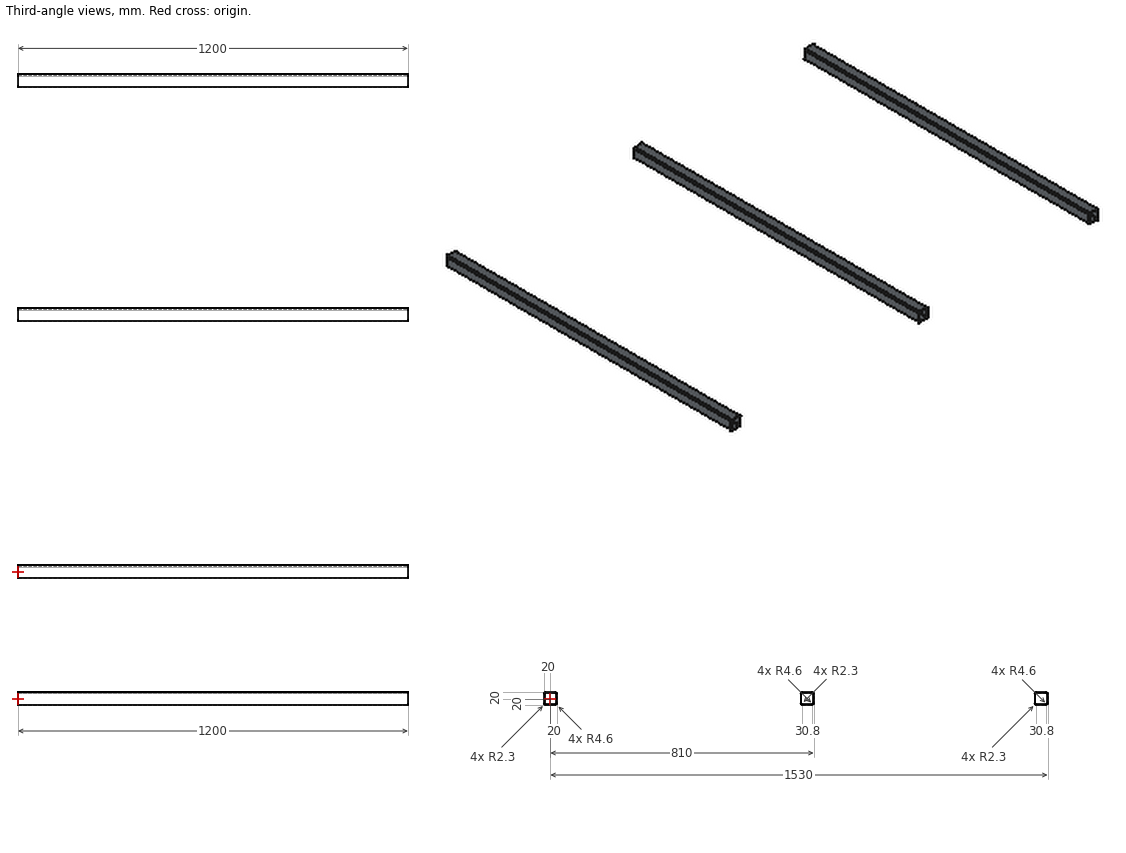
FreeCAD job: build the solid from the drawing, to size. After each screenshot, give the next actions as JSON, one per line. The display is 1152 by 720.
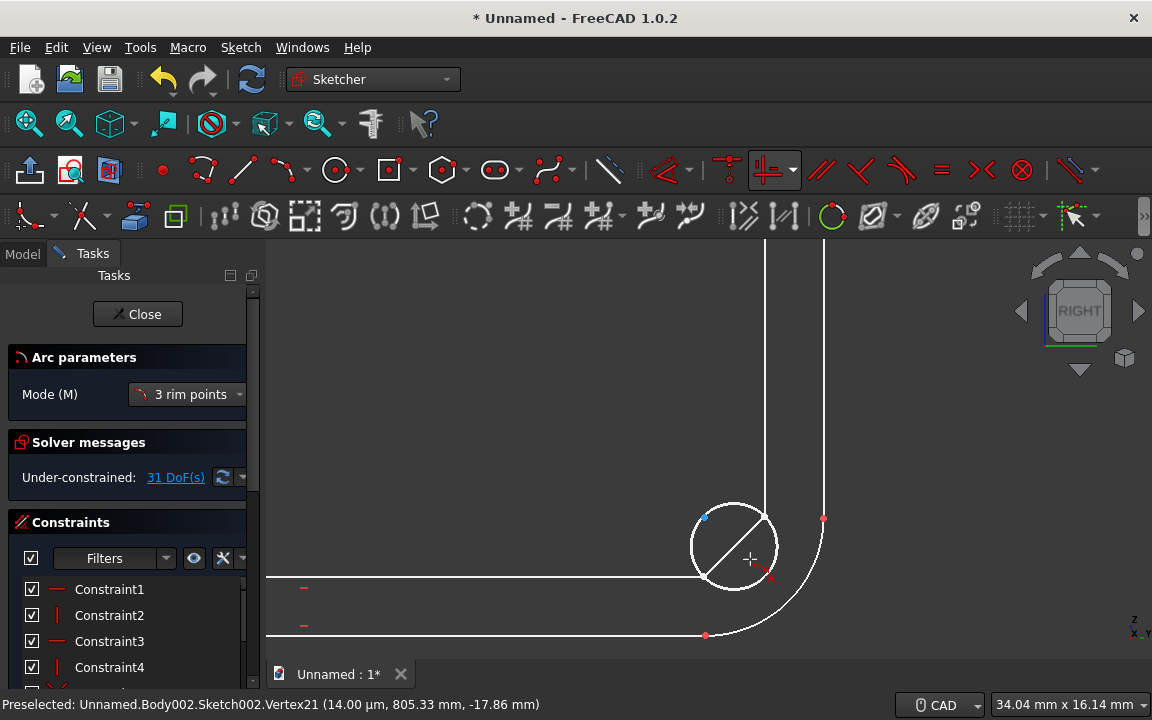
{"action": "left_click", "coordinate": [748, 555]}
{"action": "key", "text": "Escape"}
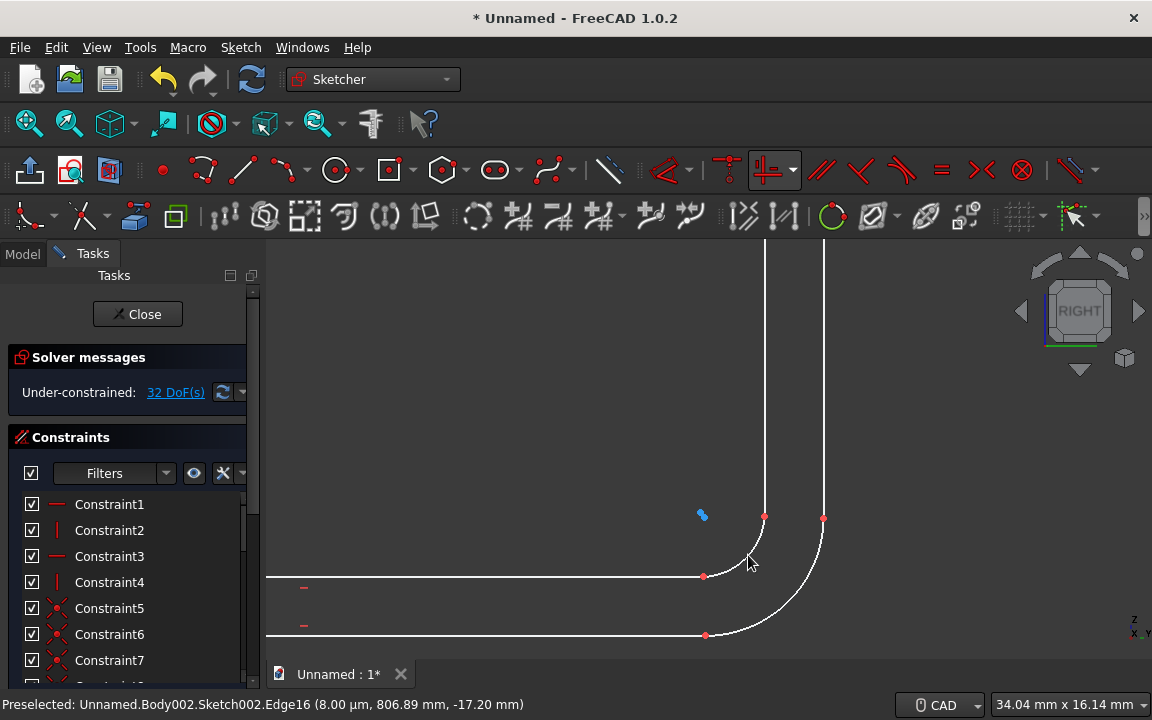
{"action": "scroll", "coordinate": [750, 559], "scroll_direction": "down", "scroll_amount": 7}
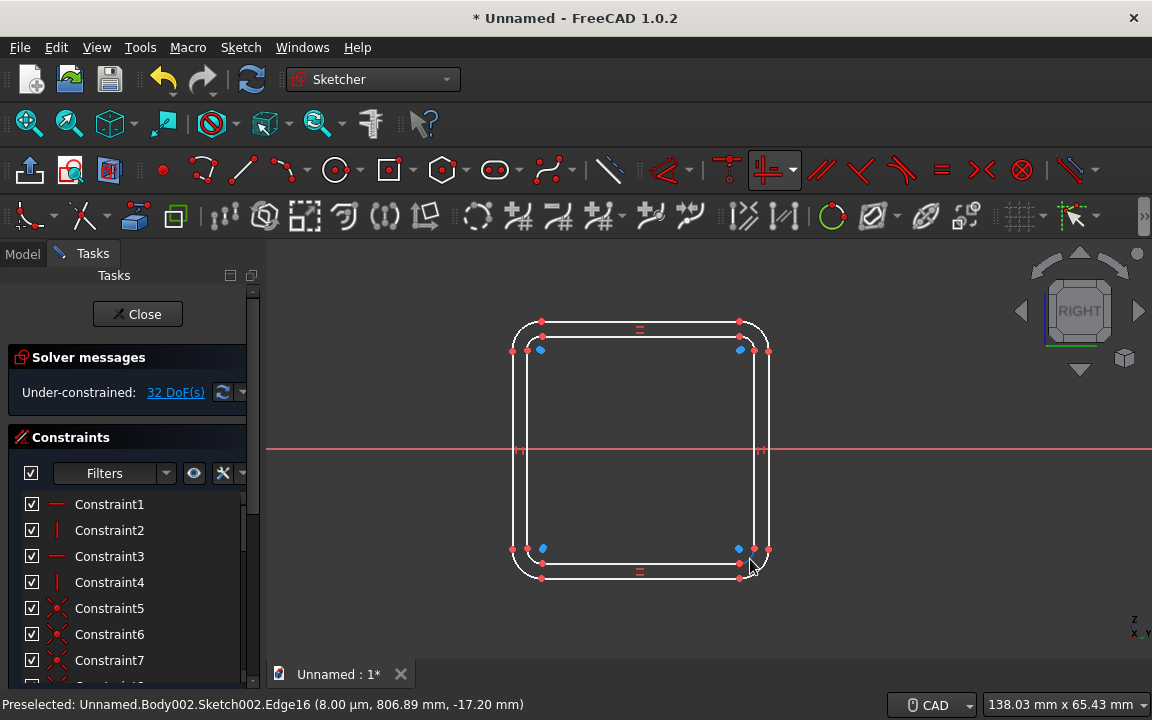
{"action": "left_click", "coordinate": [601, 579]}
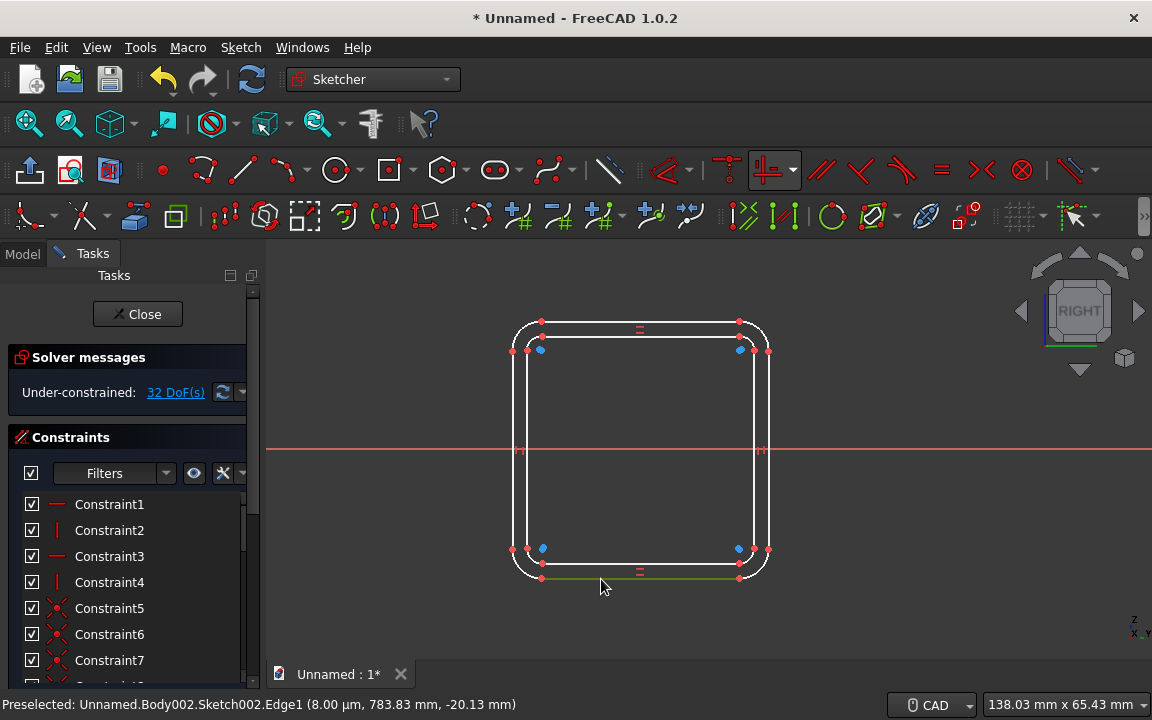
{"action": "left_click", "coordinate": [753, 575]}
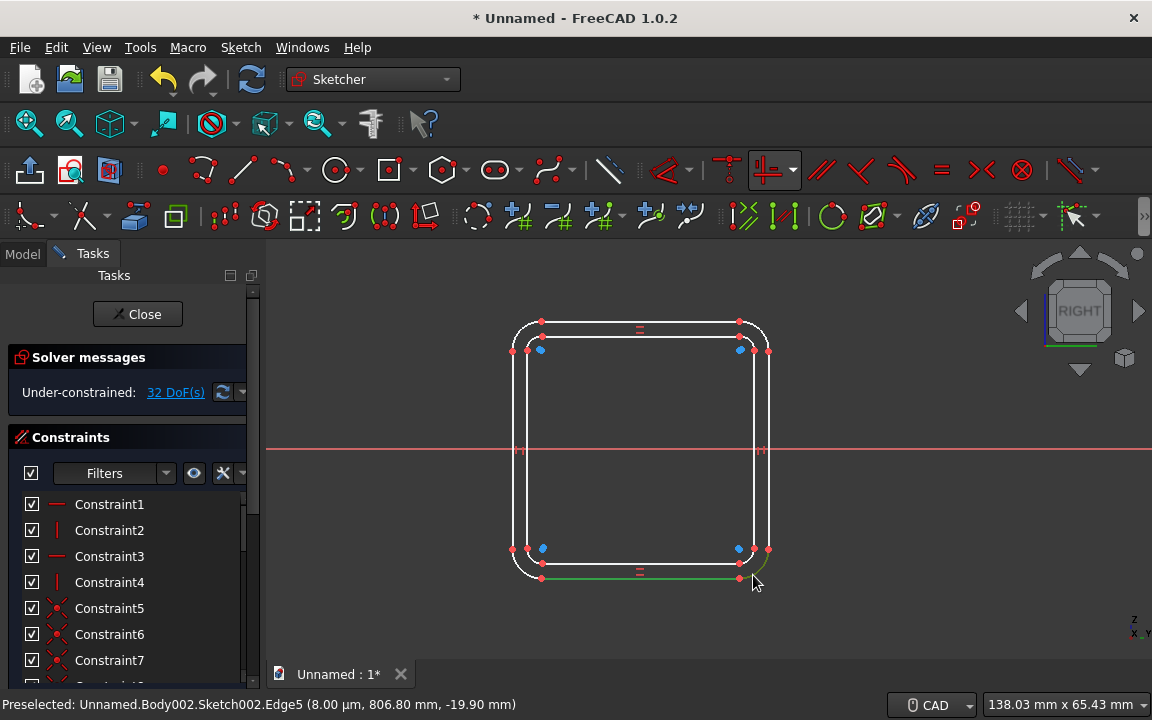
{"action": "left_click", "coordinate": [902, 170]}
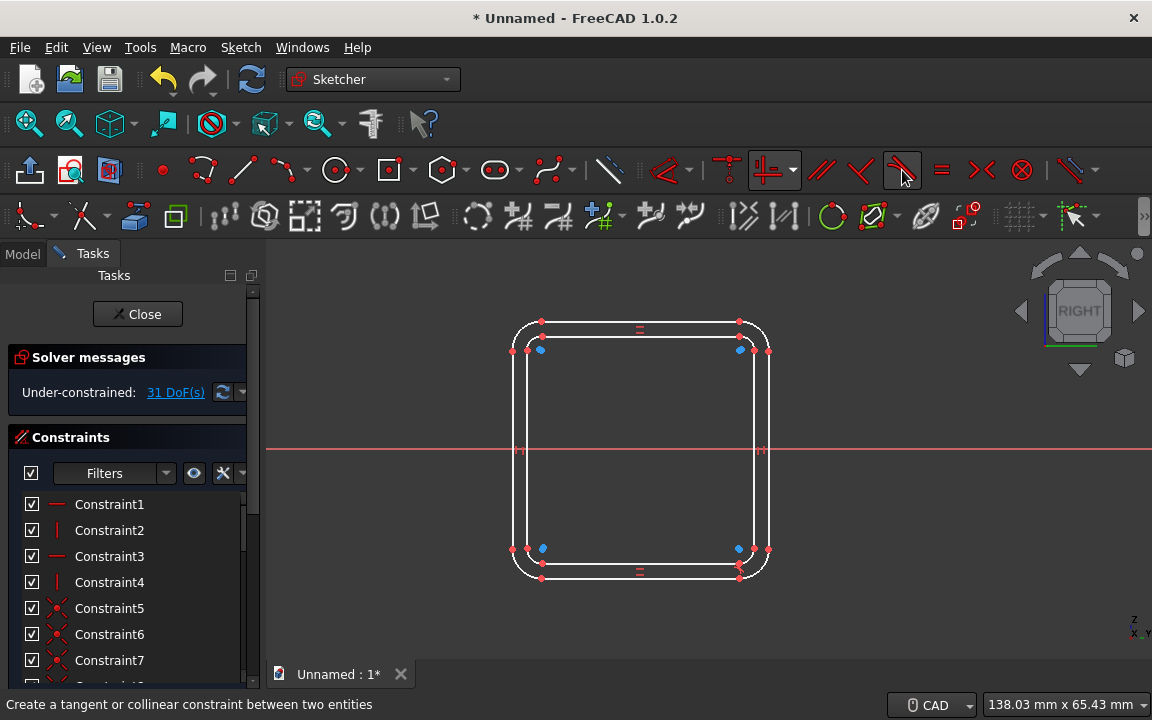
{"action": "left_click", "coordinate": [601, 579]}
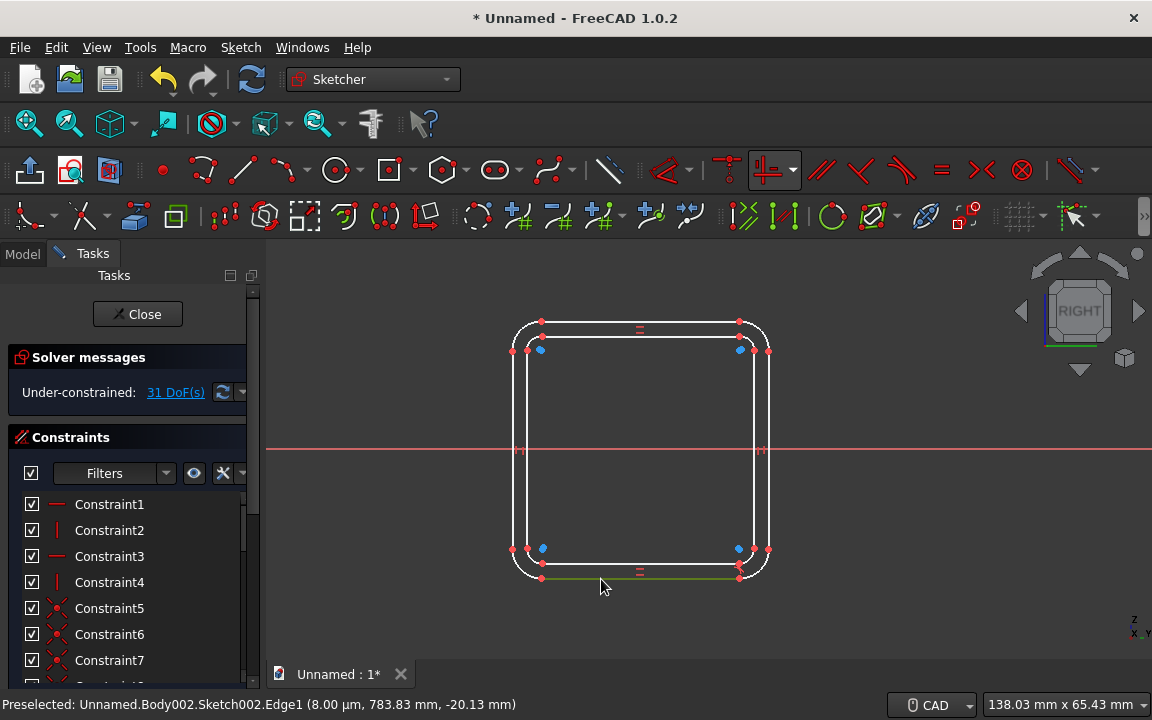
{"action": "left_click", "coordinate": [516, 563]}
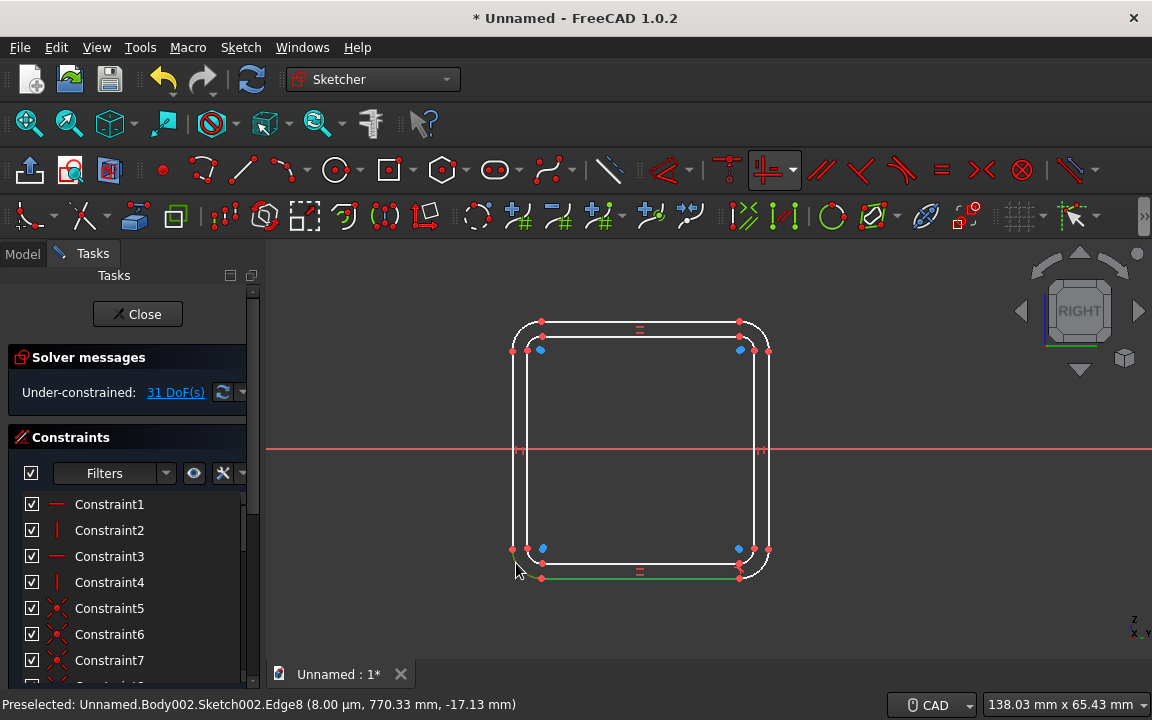
{"action": "key", "text": "t"}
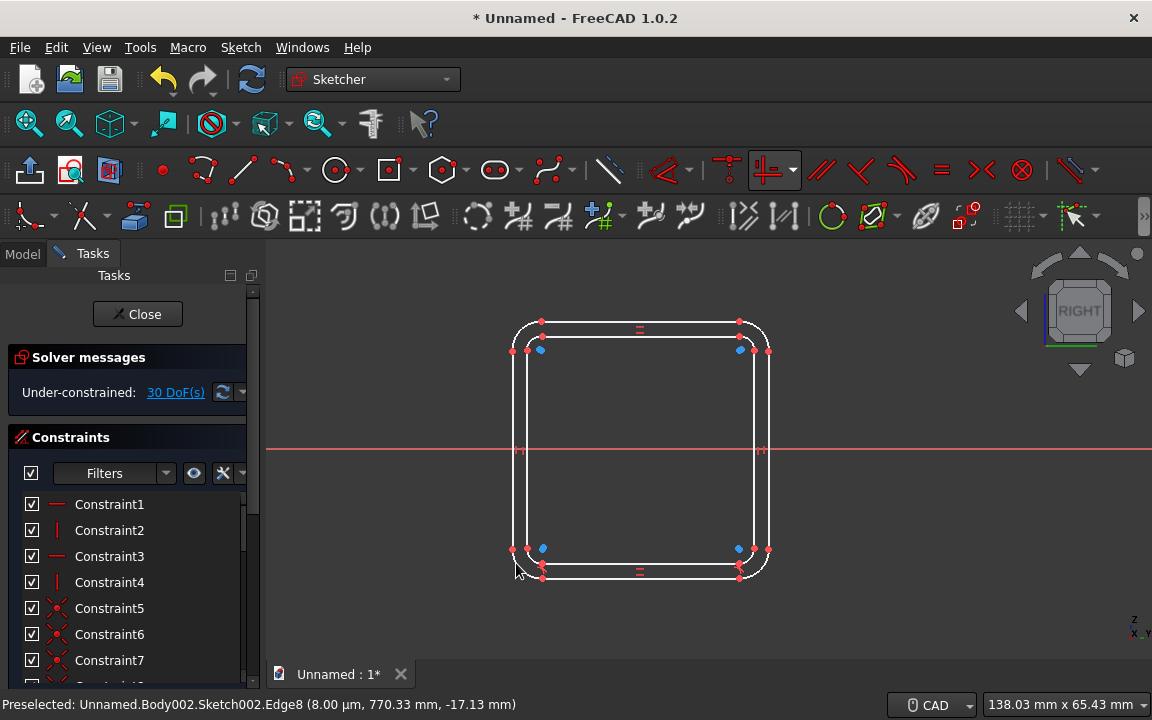
{"action": "left_click", "coordinate": [769, 490]}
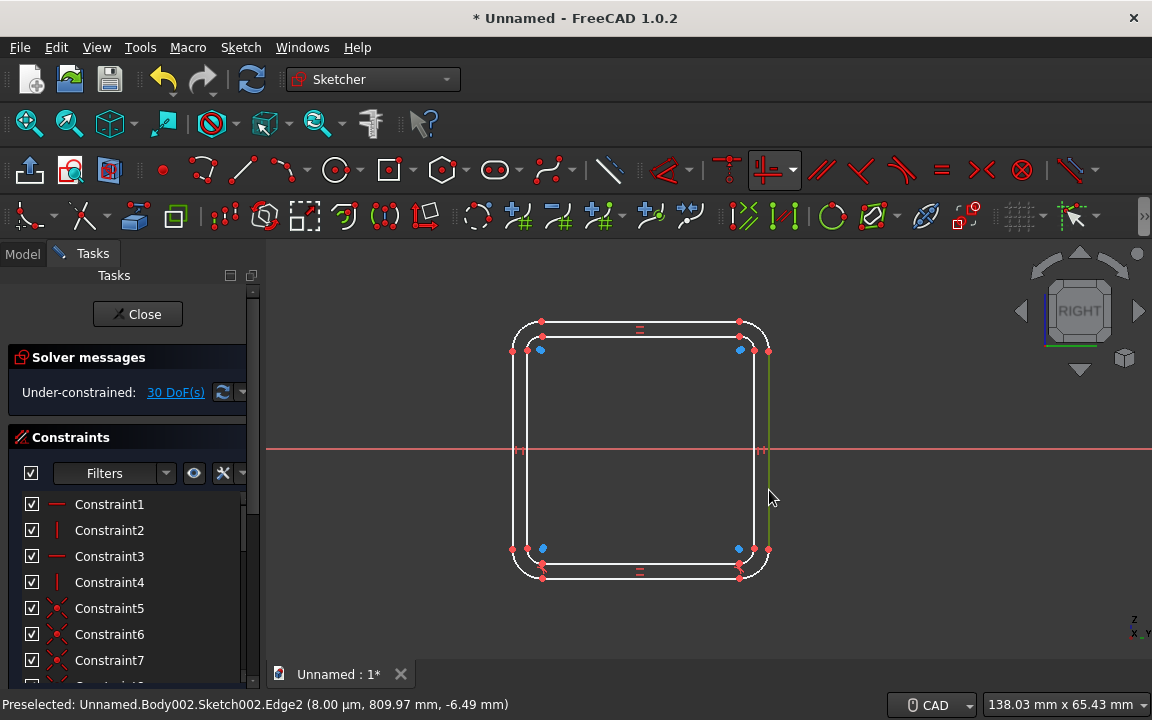
{"action": "left_click", "coordinate": [753, 575]}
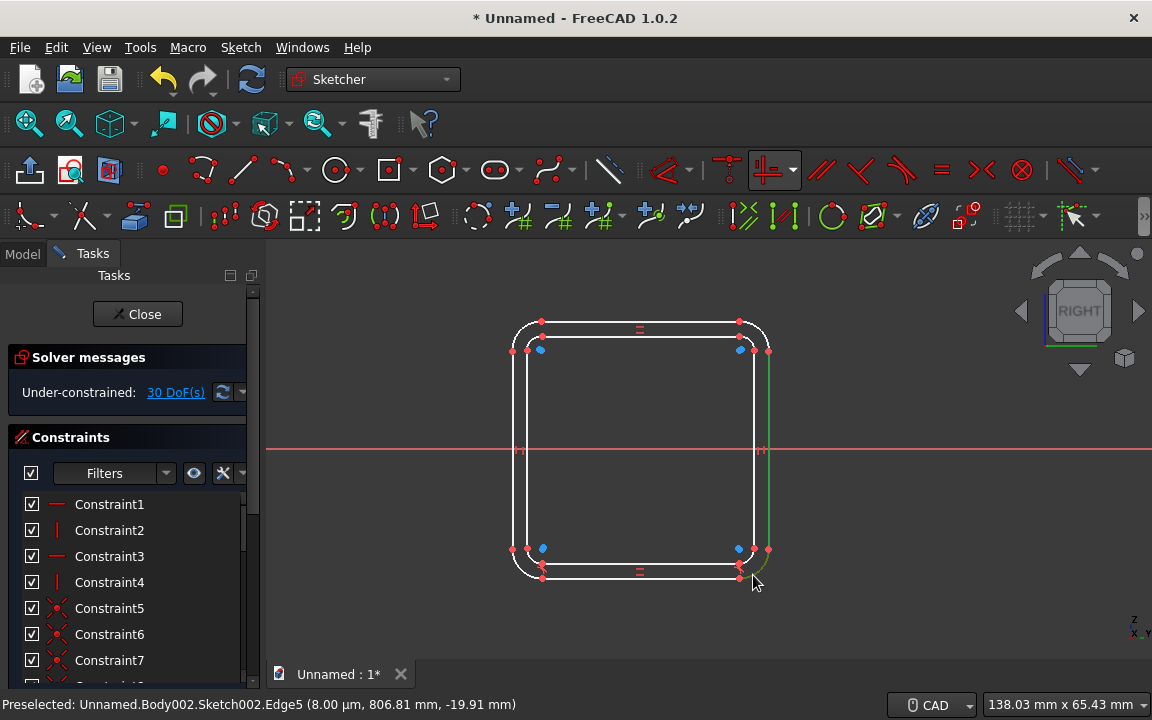
{"action": "left_click", "coordinate": [902, 170]}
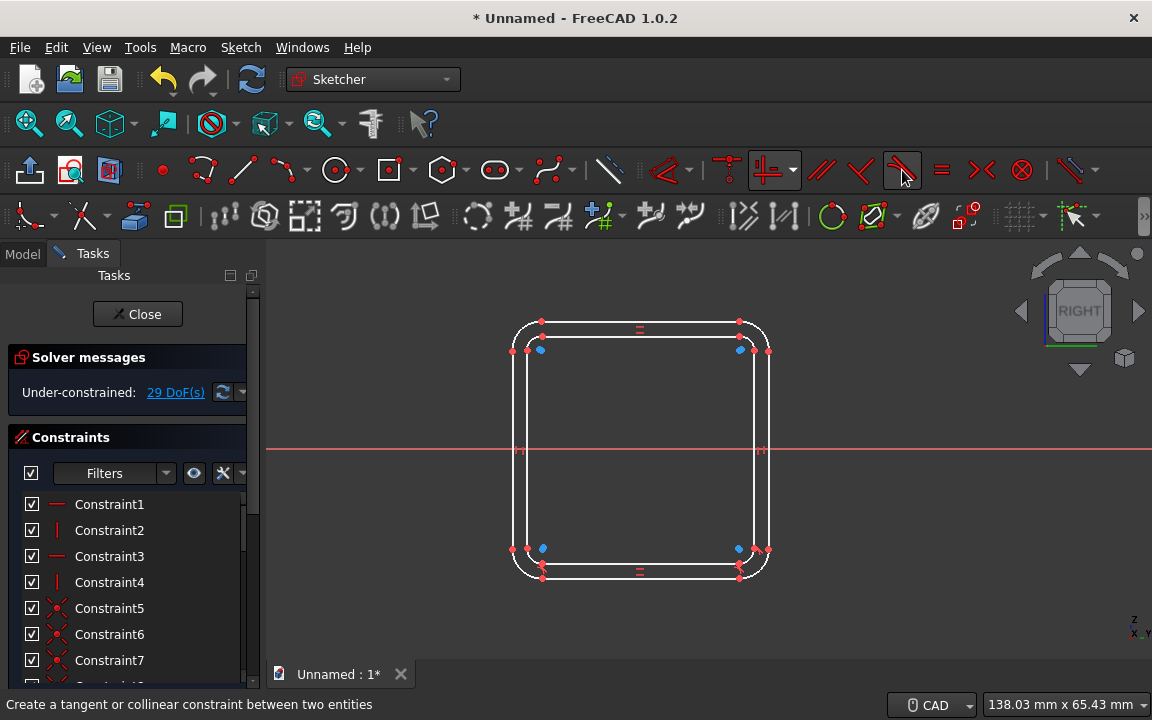
{"action": "left_click", "coordinate": [769, 490]}